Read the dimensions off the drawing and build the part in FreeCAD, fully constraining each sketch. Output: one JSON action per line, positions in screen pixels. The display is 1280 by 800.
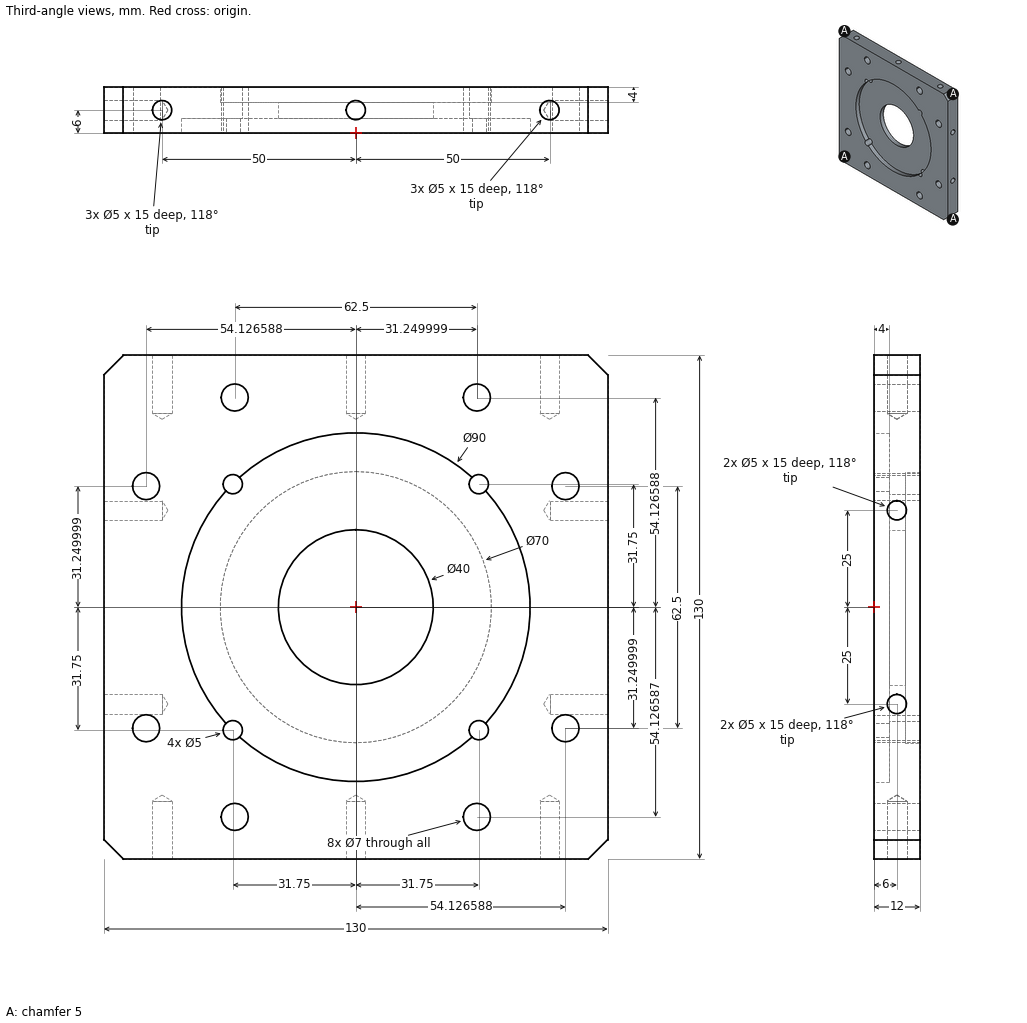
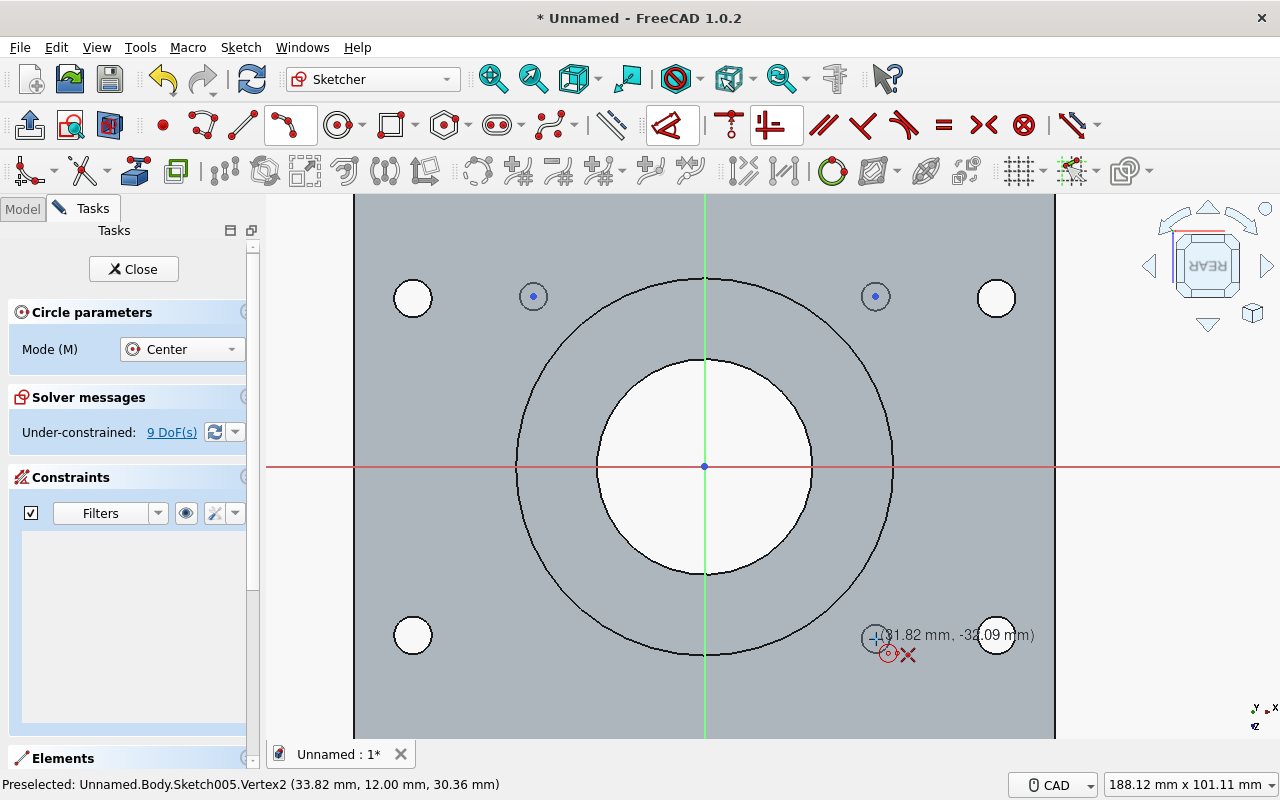
{"action": "scroll", "coordinate": [534, 638], "scroll_direction": "up", "scroll_amount": 3}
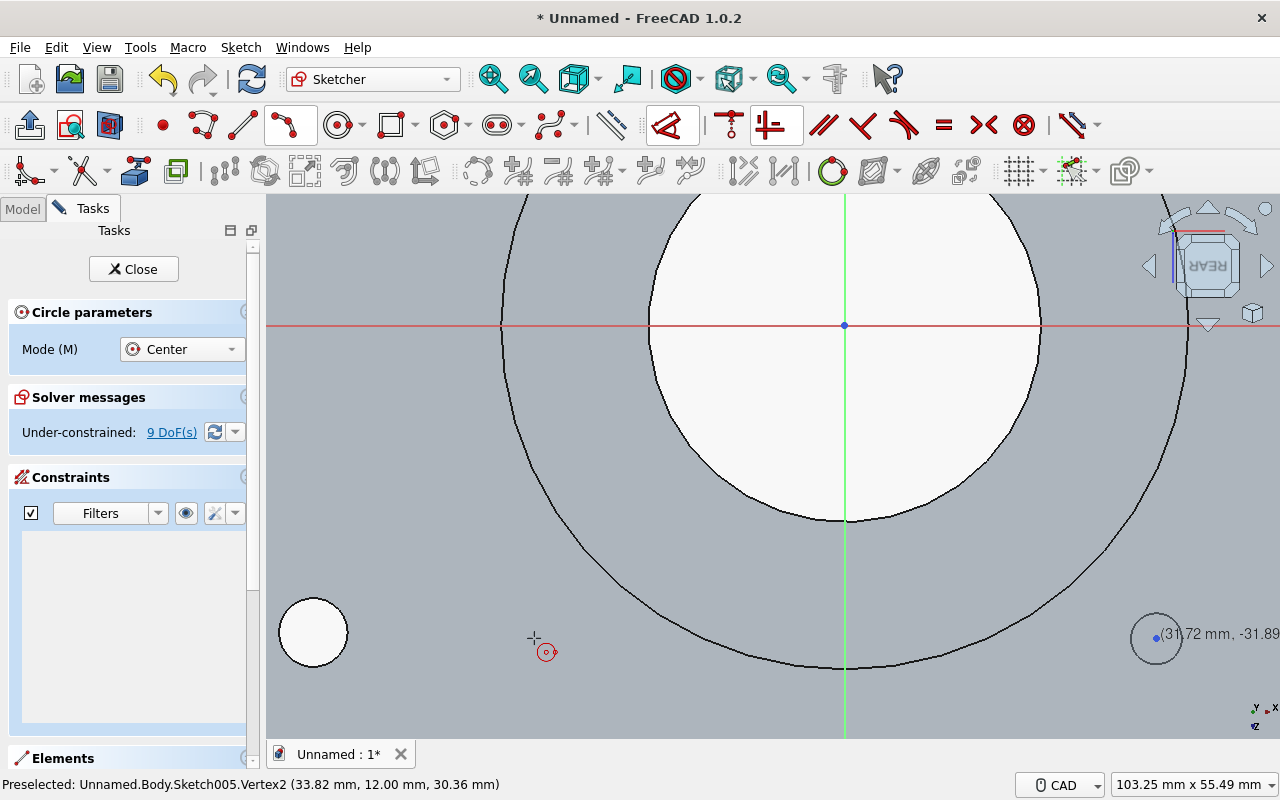
{"action": "left_click", "coordinate": [533, 637]}
{"action": "left_click", "coordinate": [550, 620]}
{"action": "key", "text": "Escape"}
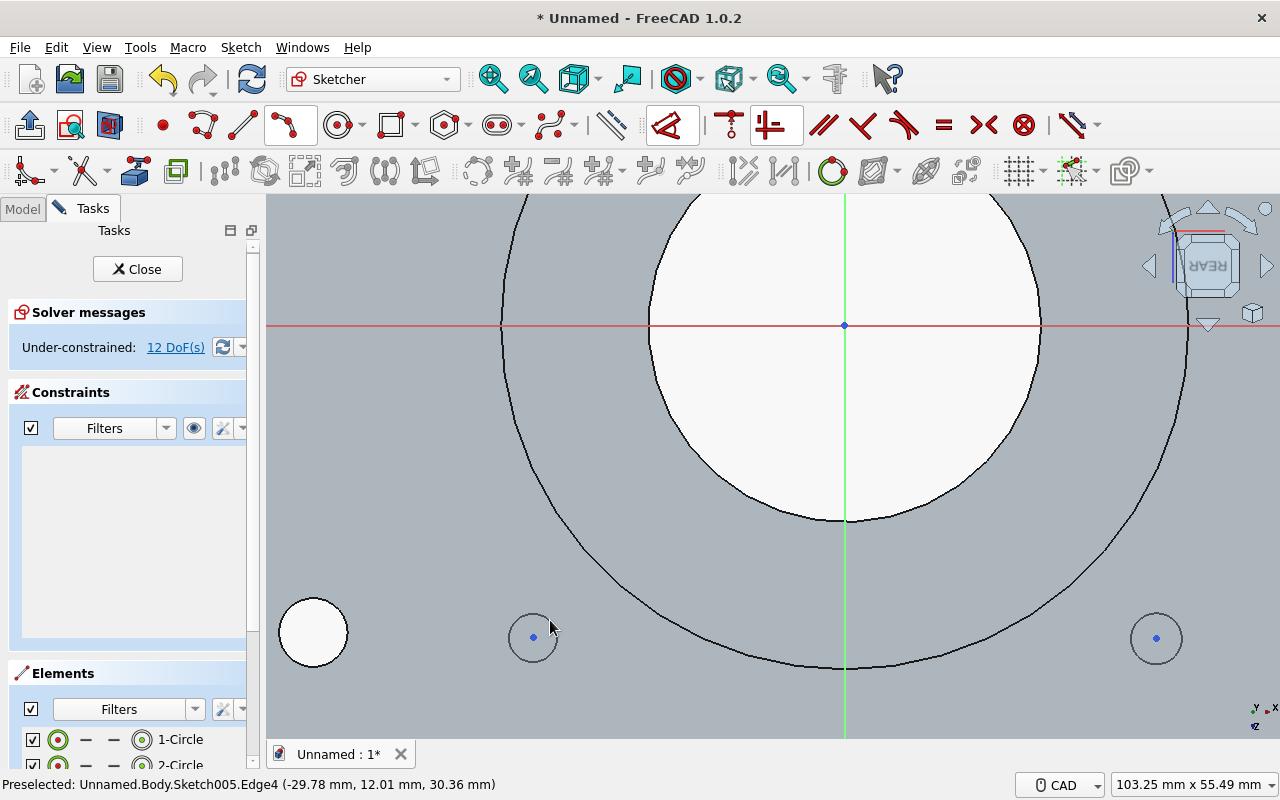
{"action": "scroll", "coordinate": [534, 638], "scroll_direction": "down", "scroll_amount": 3}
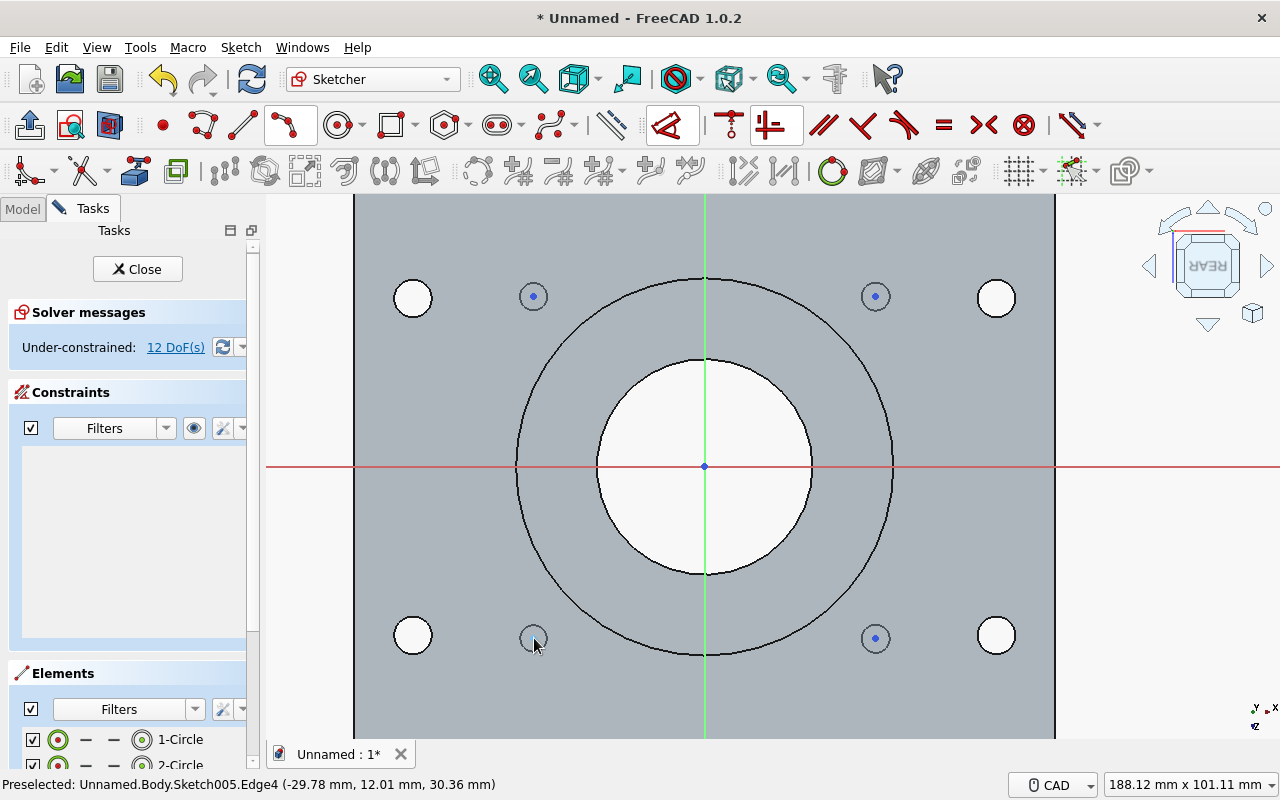
{"action": "left_click", "coordinate": [543, 287]}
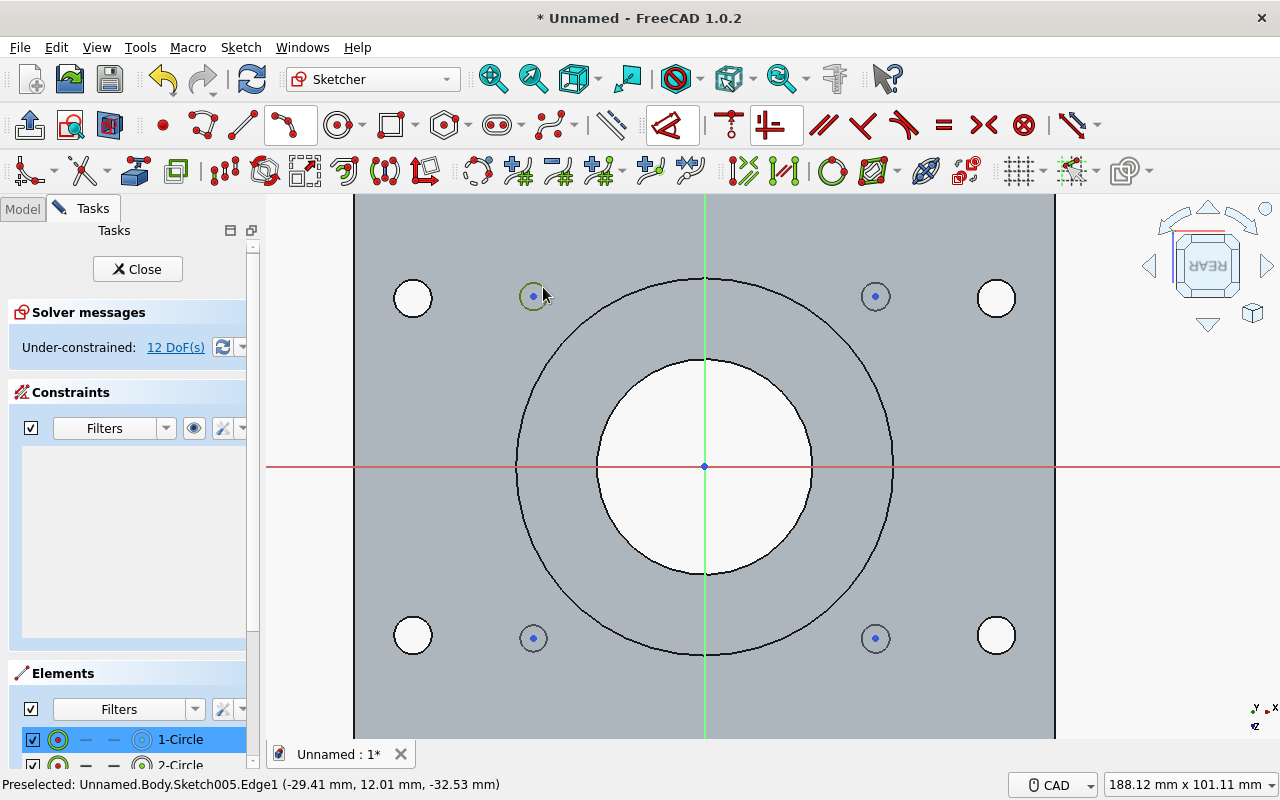
{"action": "left_click", "coordinate": [886, 287]}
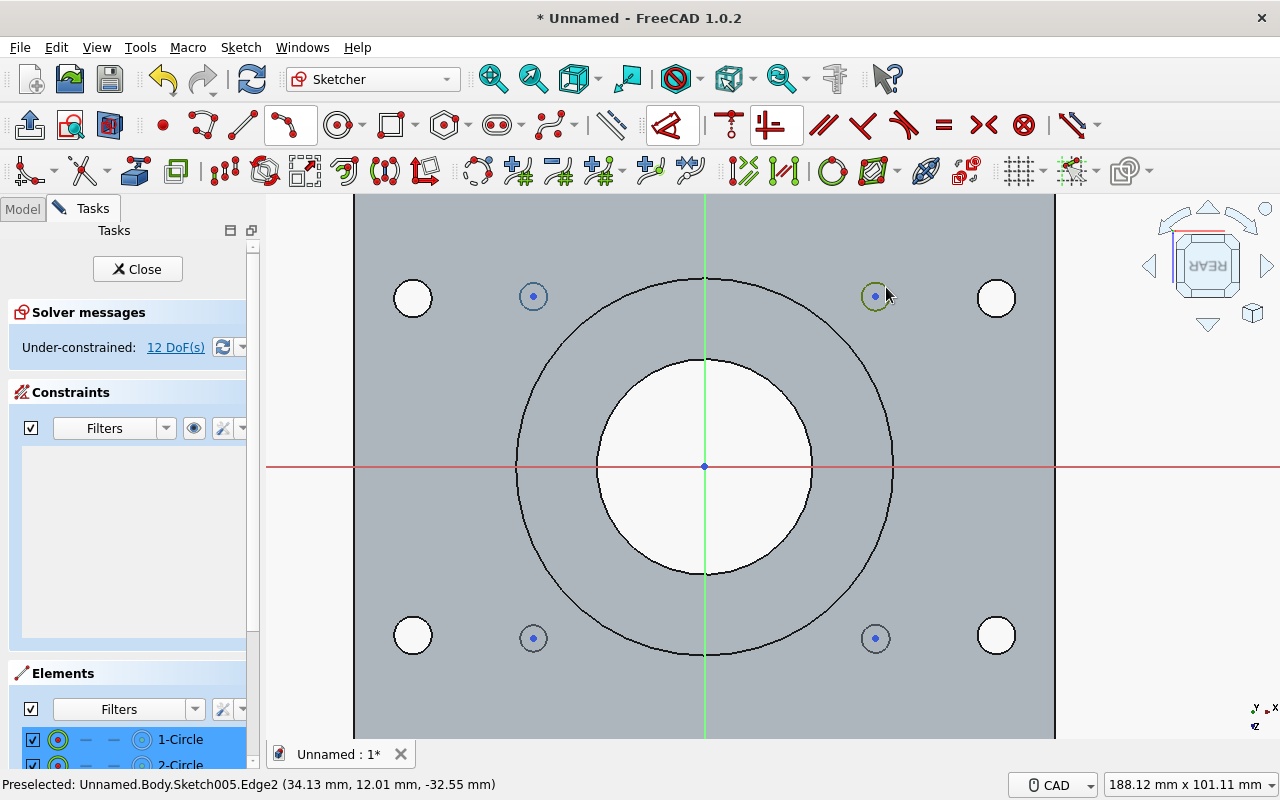
{"action": "left_click", "coordinate": [886, 629]}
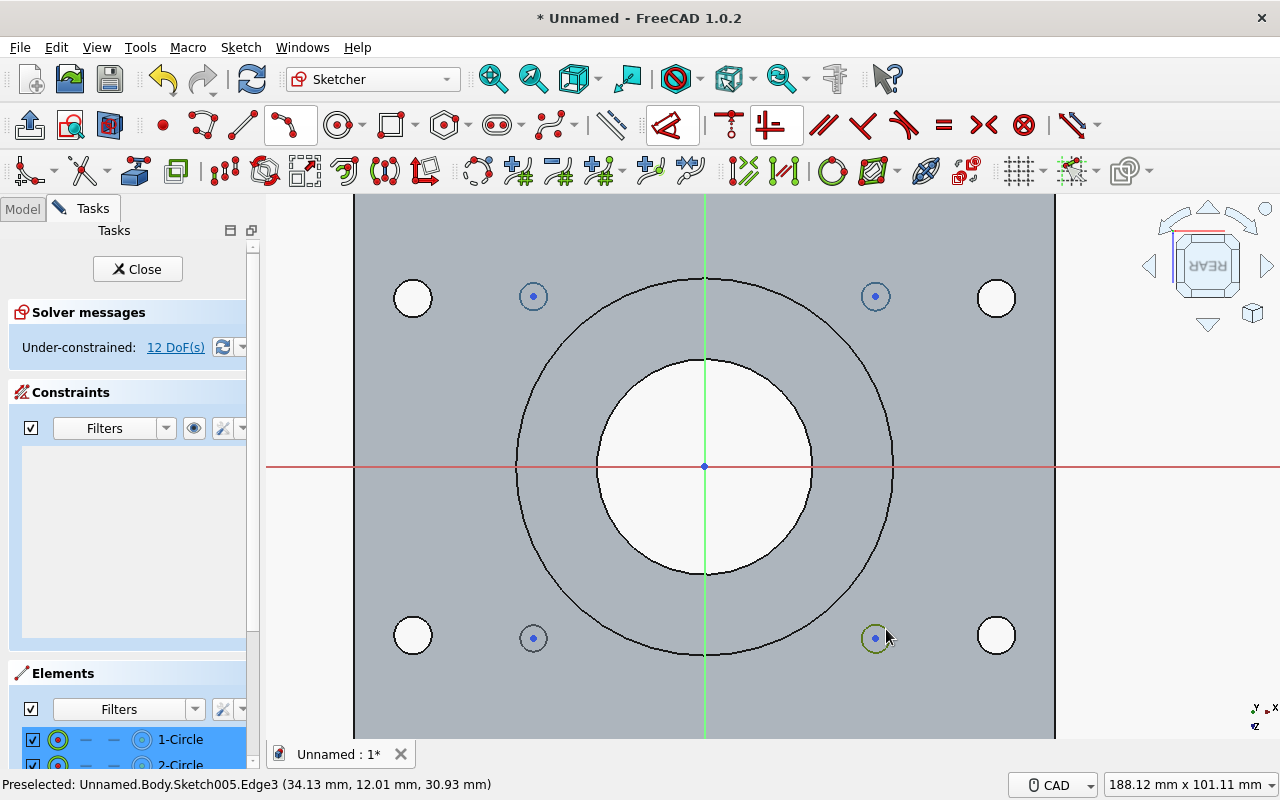
{"action": "left_click", "coordinate": [543, 629]}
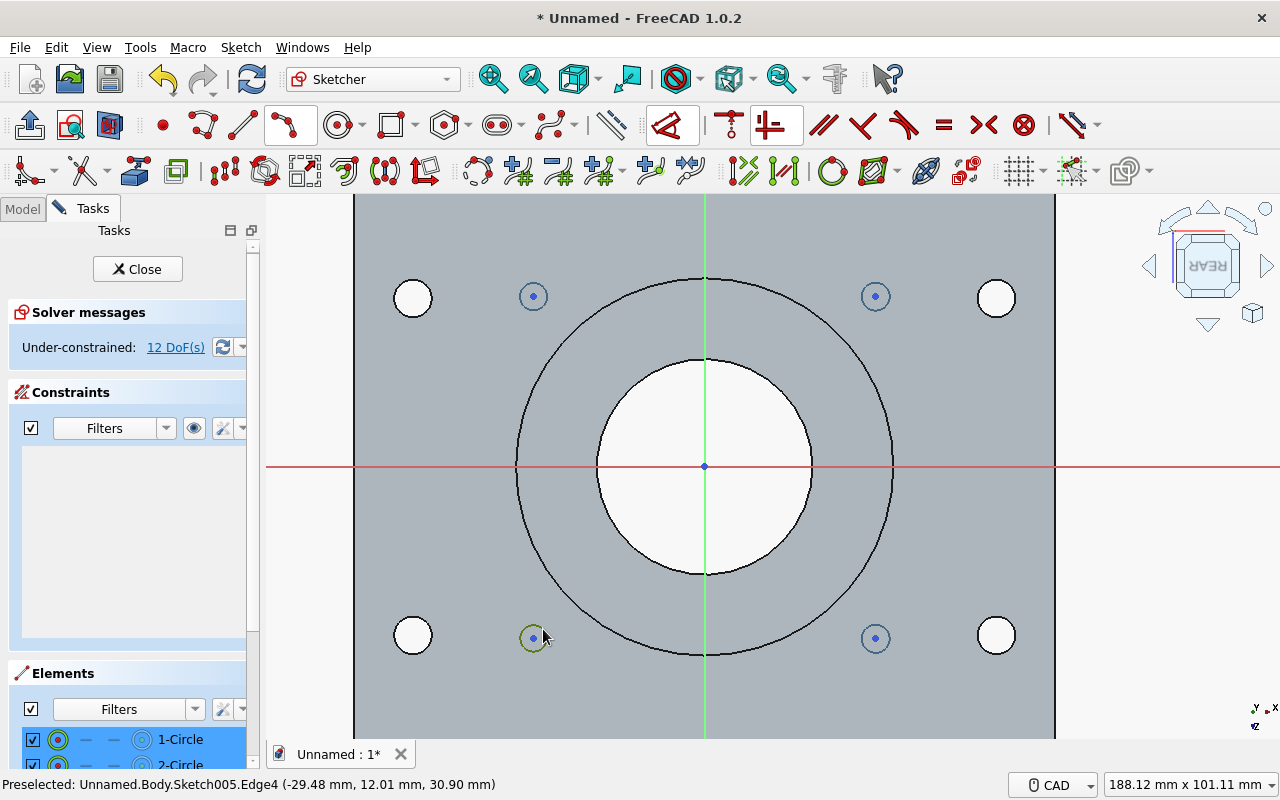
{"action": "key", "text": "e"}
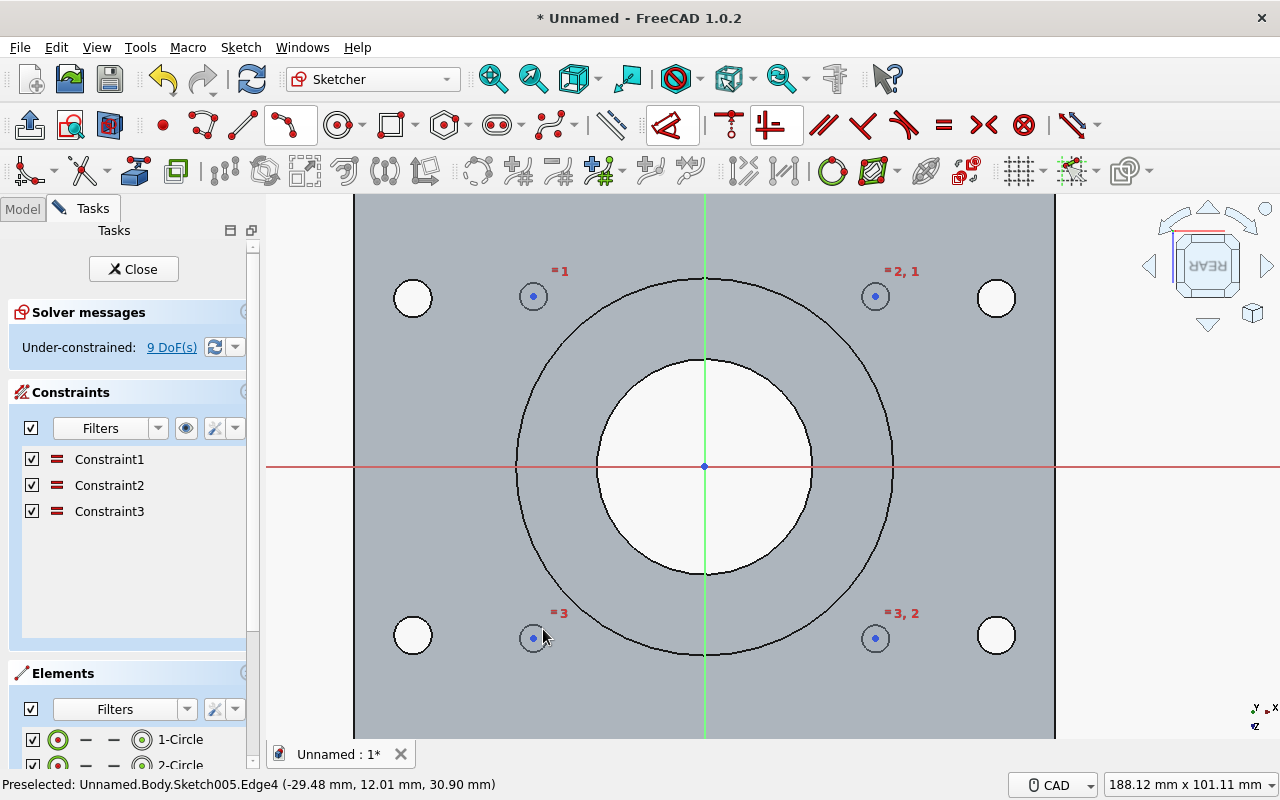
{"action": "left_click", "coordinate": [534, 297]}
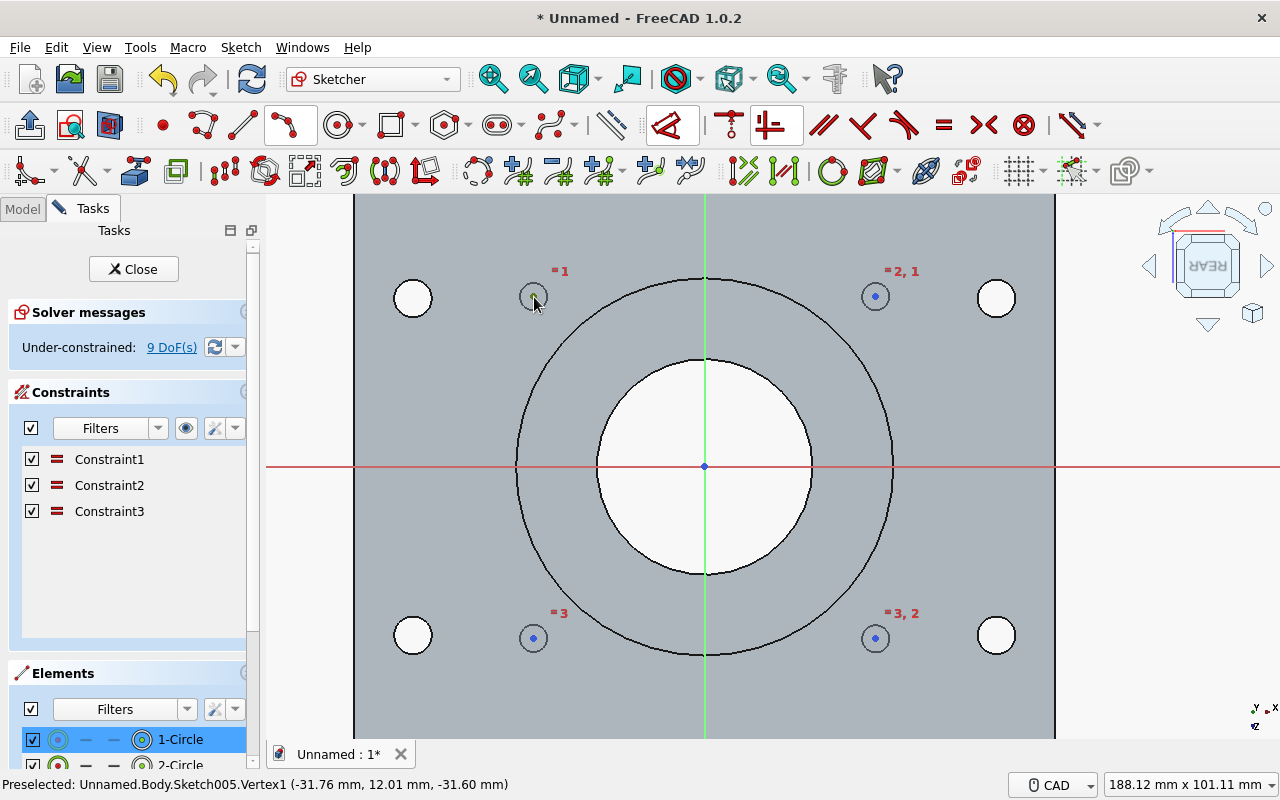
{"action": "left_click", "coordinate": [876, 297]}